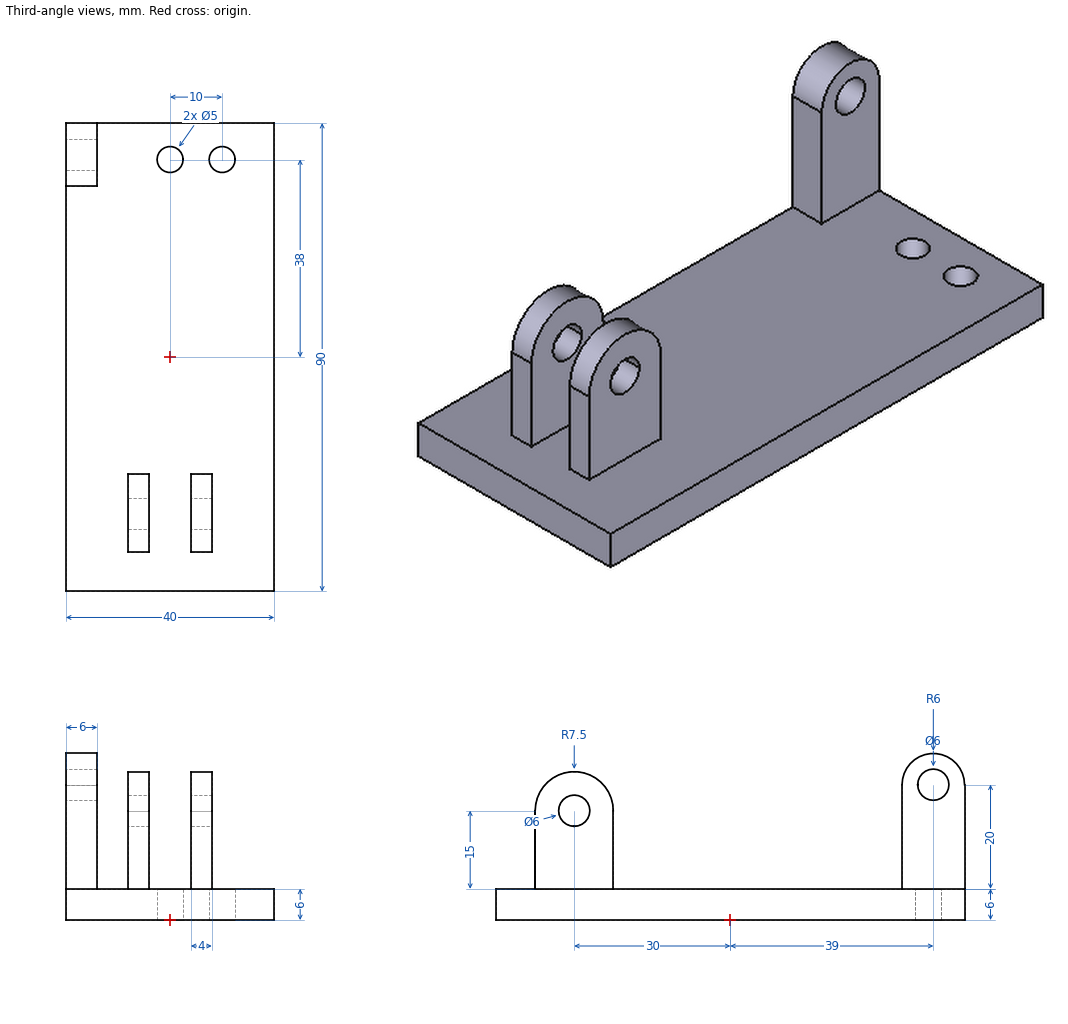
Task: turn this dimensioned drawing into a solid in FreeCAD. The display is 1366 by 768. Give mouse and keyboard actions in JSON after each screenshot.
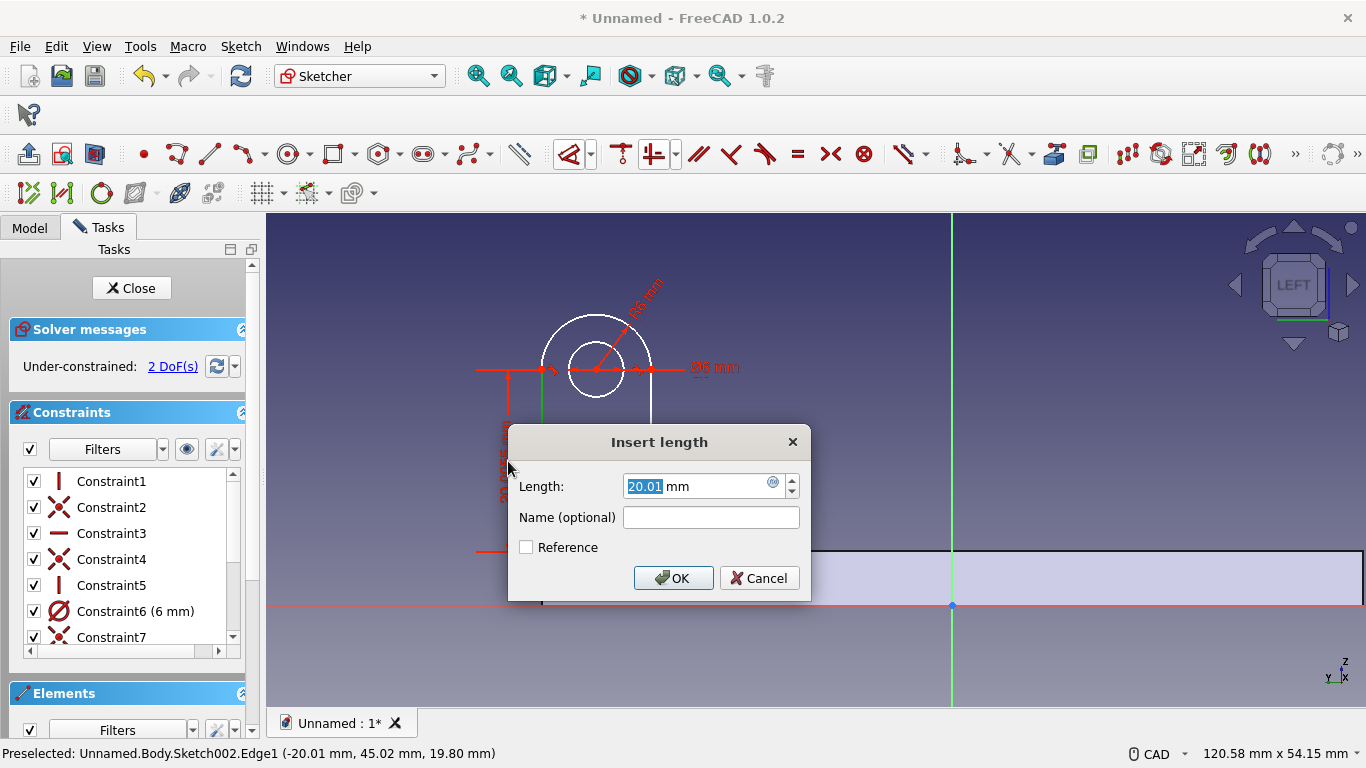
{"action": "type", "text": "20"}
{"action": "key", "text": "Return"}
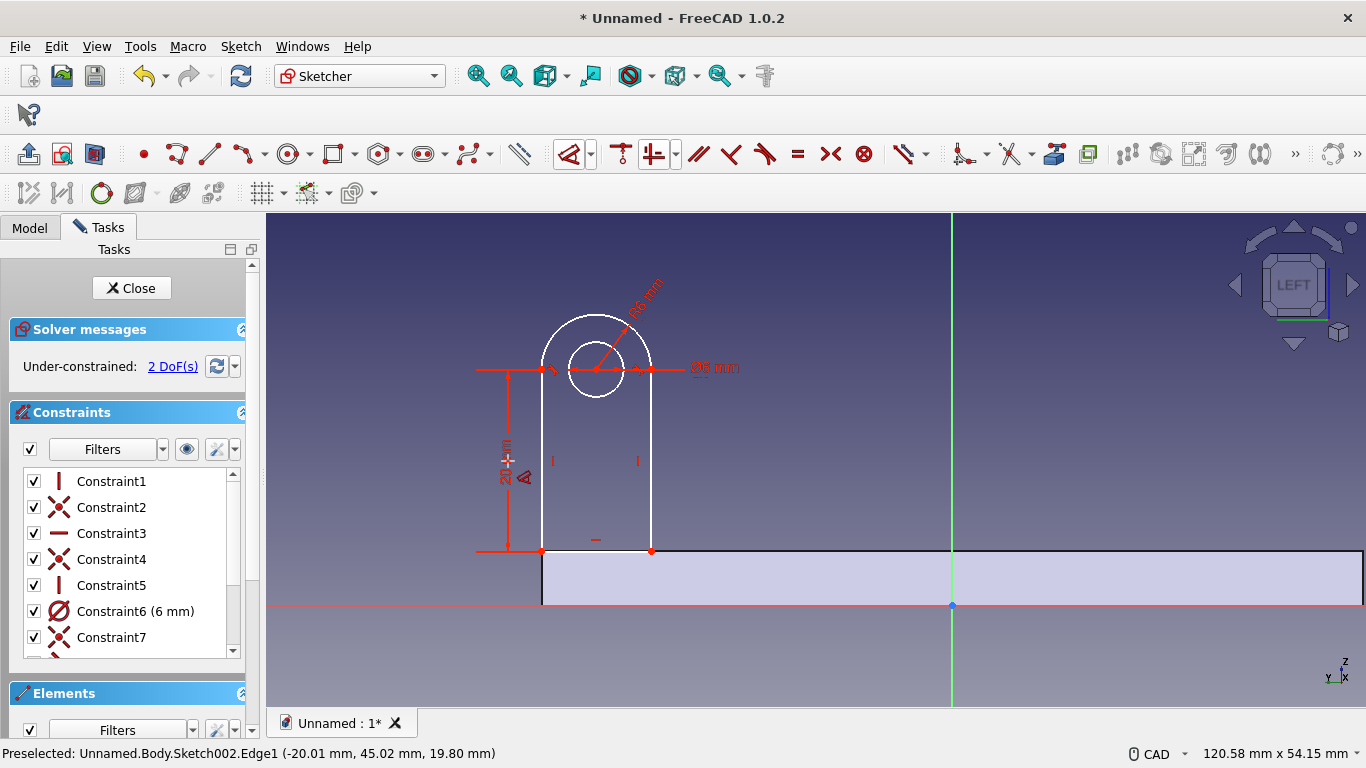
{"action": "left_click", "coordinate": [542, 552]}
{"action": "left_click", "coordinate": [508, 579]}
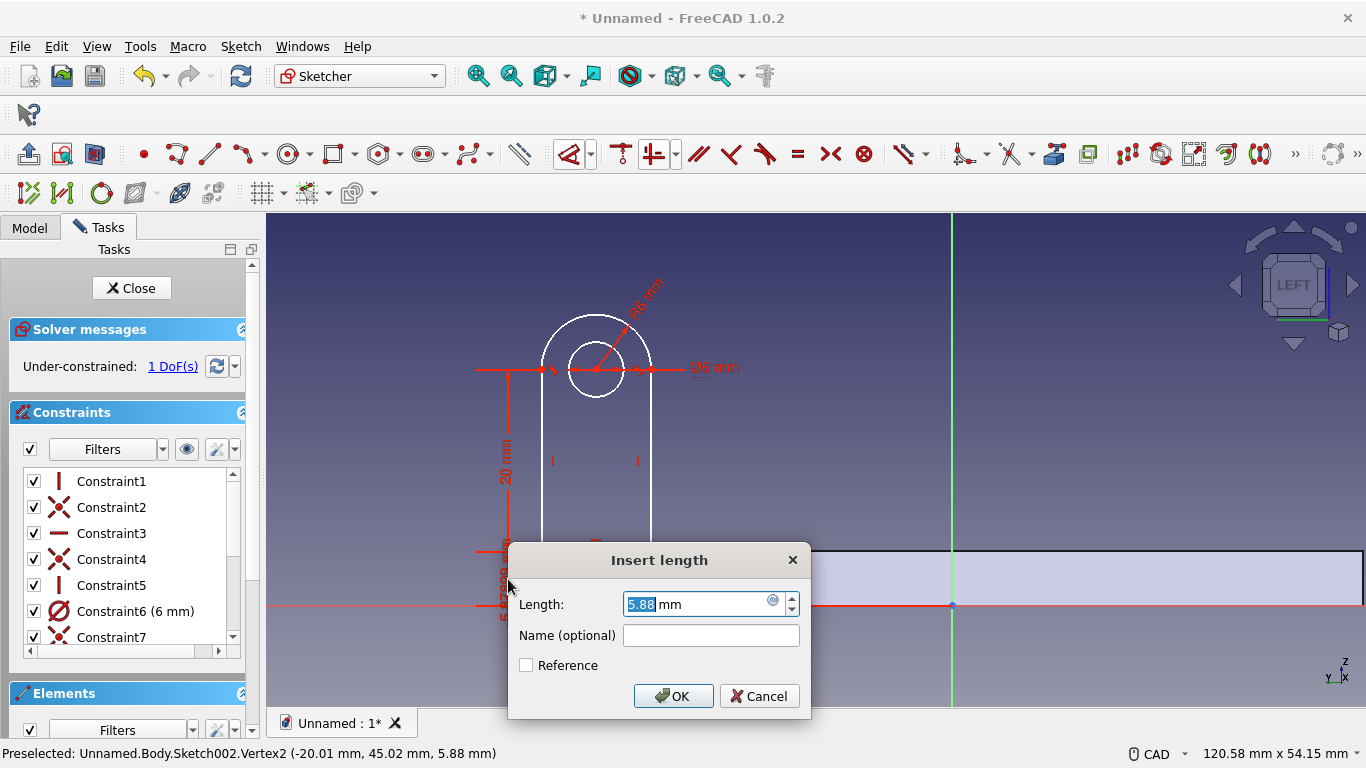
{"action": "type", "text": "6"}
{"action": "key", "text": "Return"}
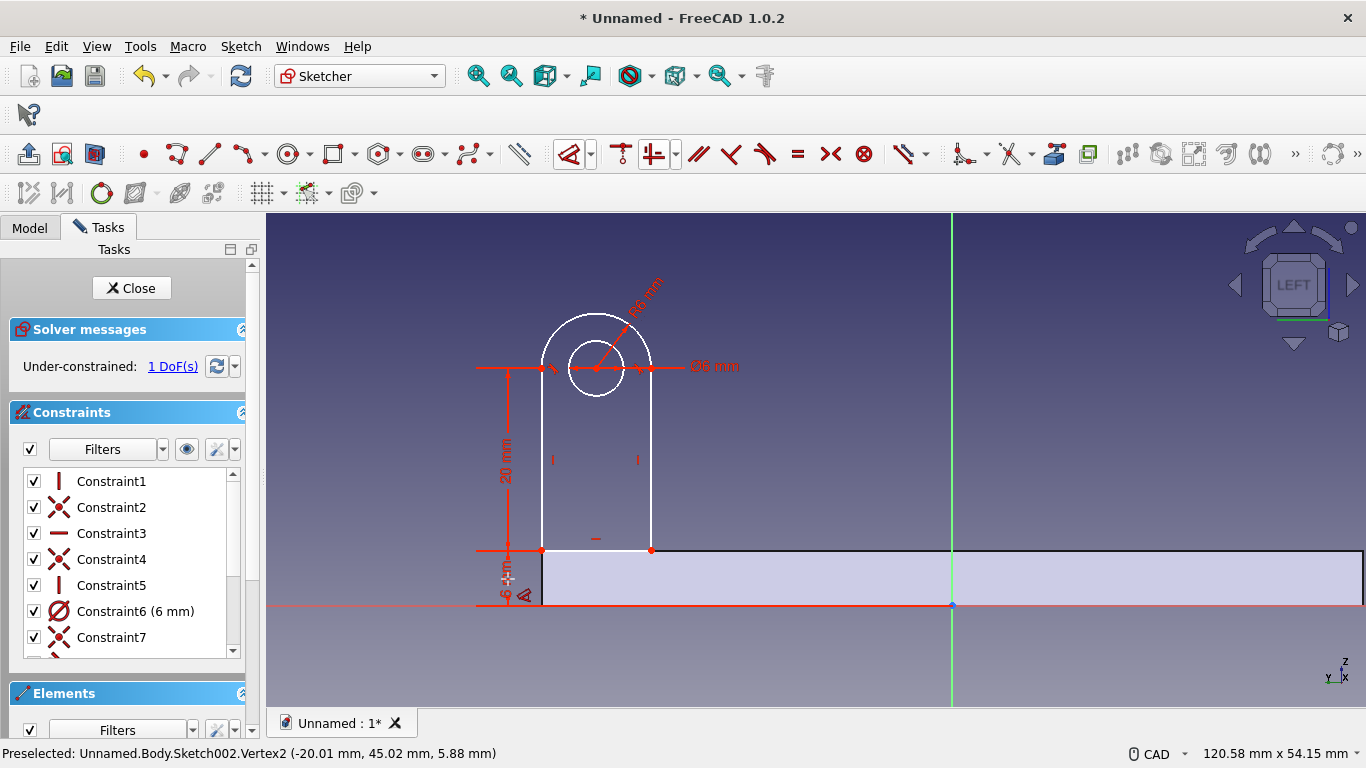
{"action": "left_click", "coordinate": [596, 368]}
{"action": "left_click", "coordinate": [774, 640]}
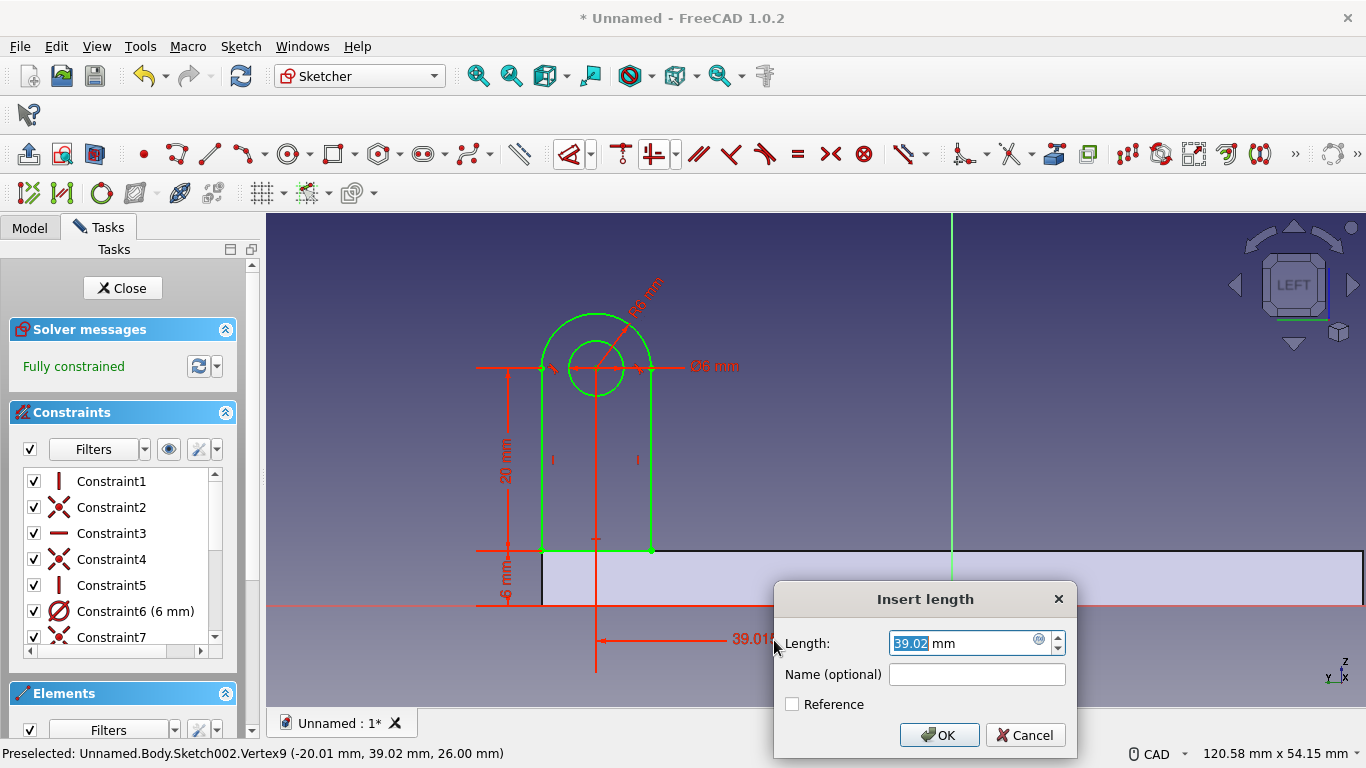
{"action": "type", "text": "39"}
{"action": "key", "text": "Return"}
{"action": "key", "text": "Escape"}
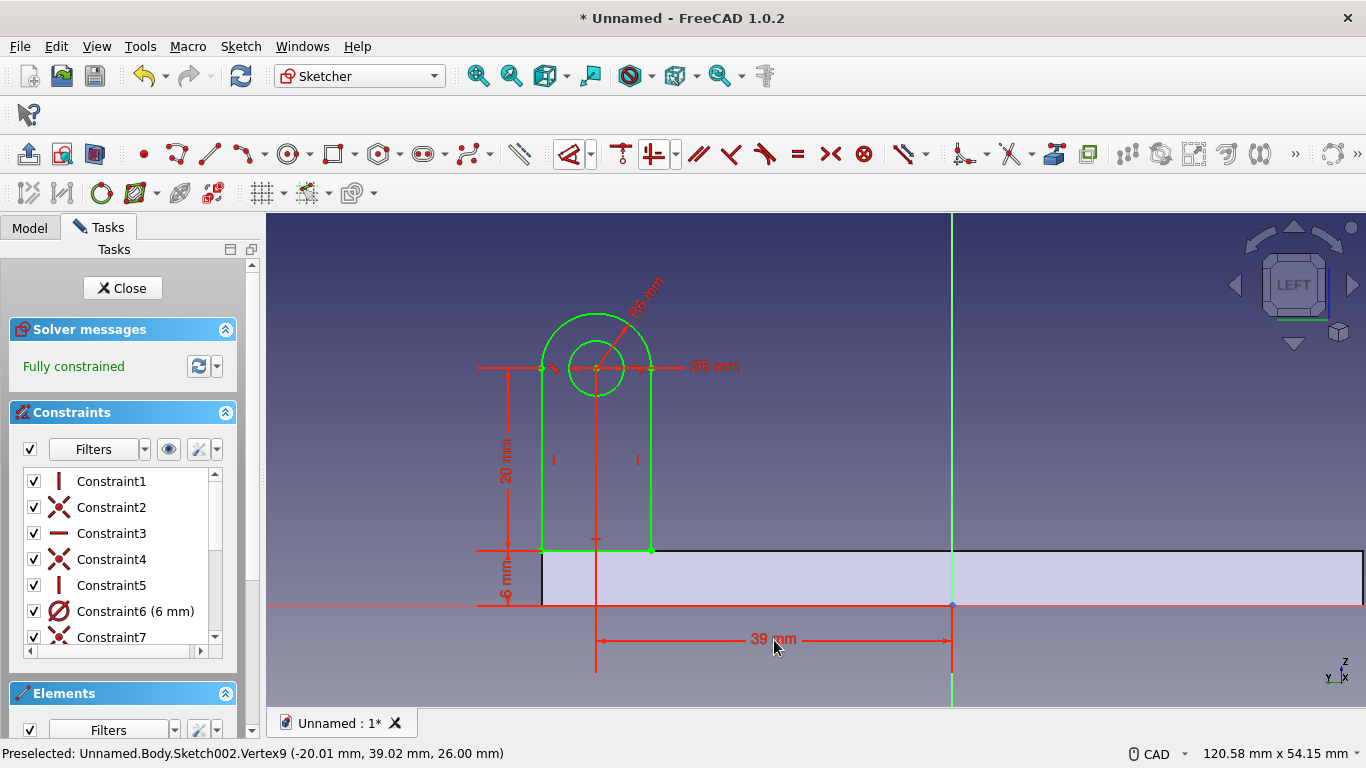
{"action": "left_click", "coordinate": [123, 288]}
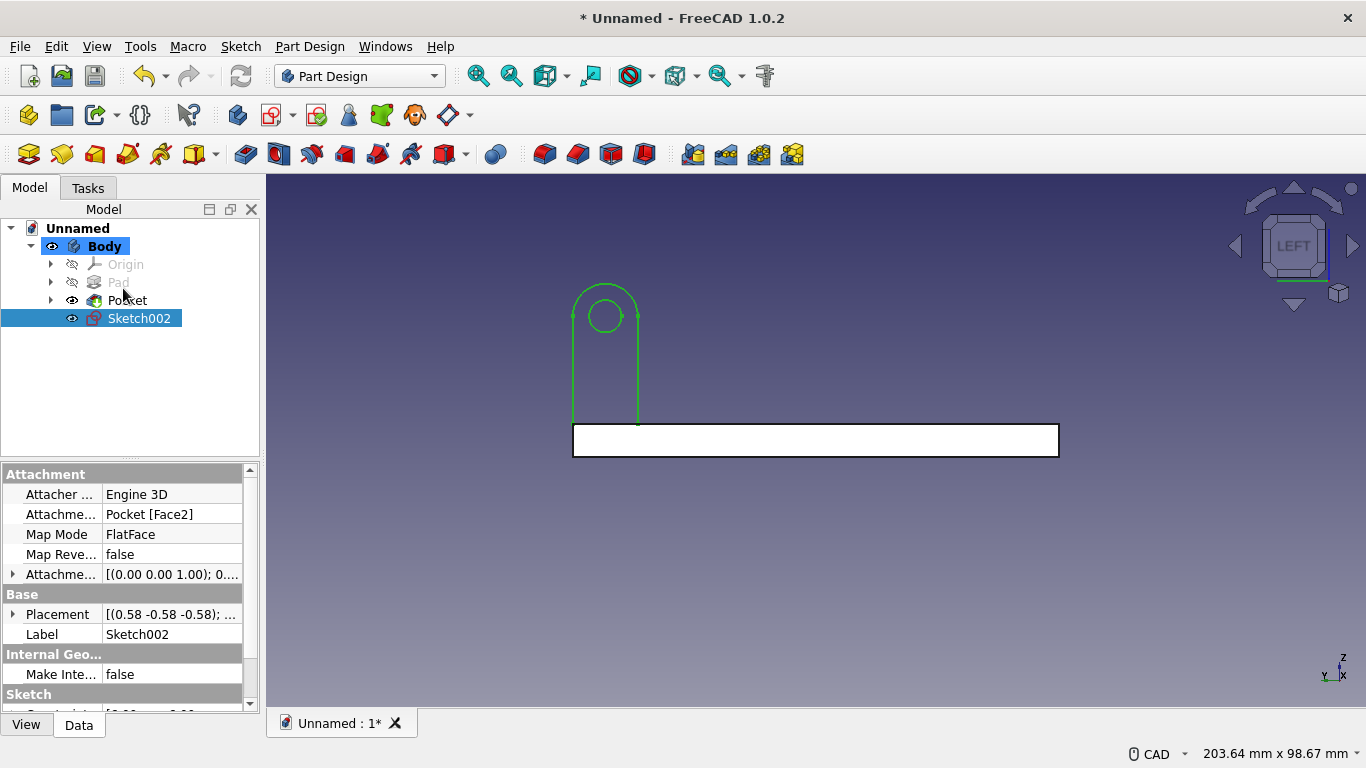
{"action": "left_click", "coordinate": [29, 154]}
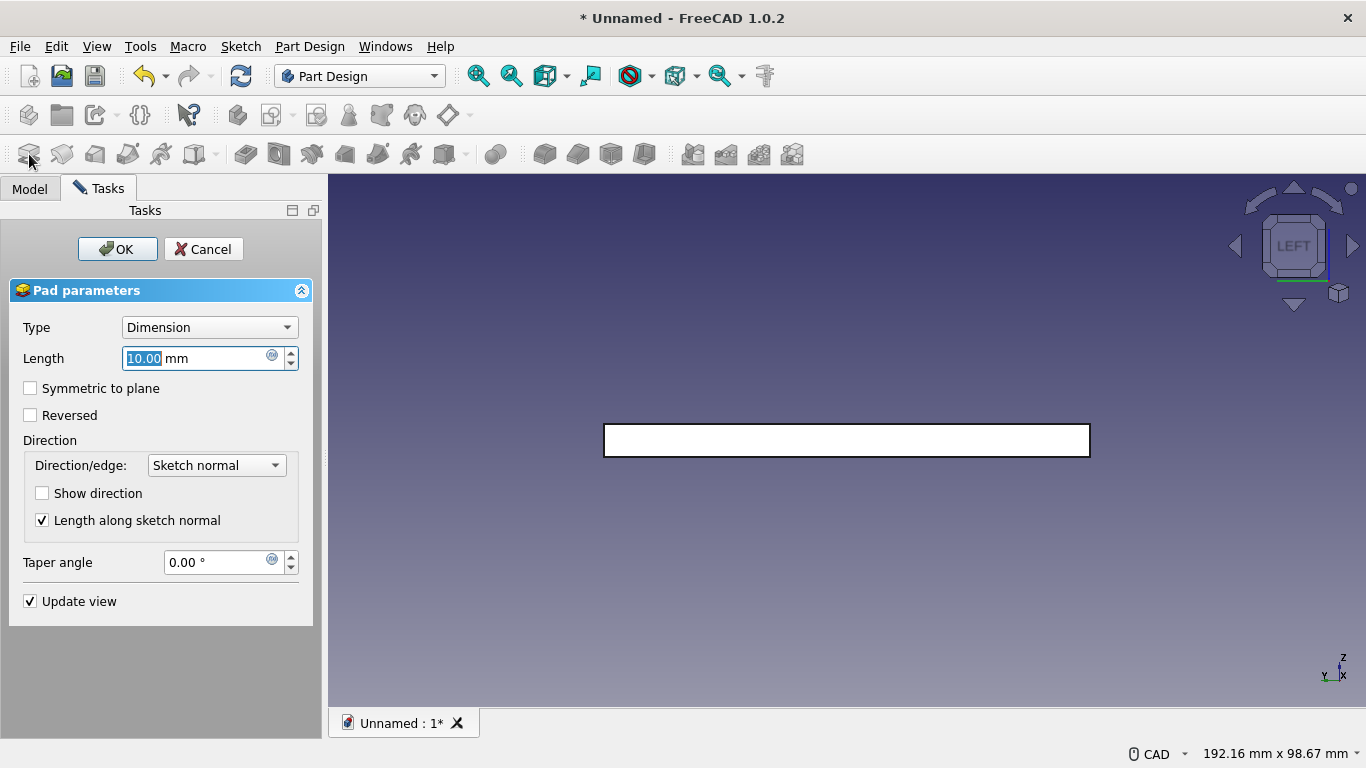
{"action": "type", "text": "6"}
{"action": "key", "text": "Tab"}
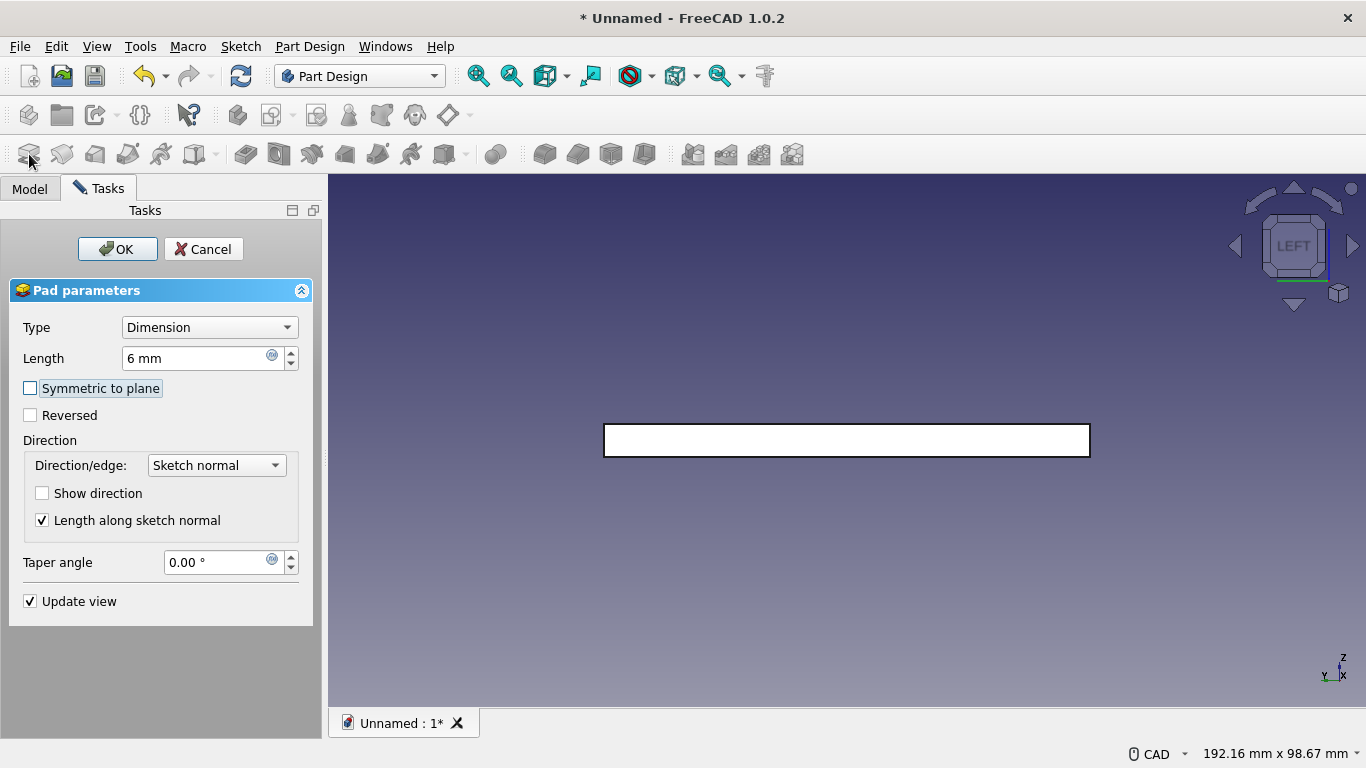
{"action": "left_click", "coordinate": [31, 415]}